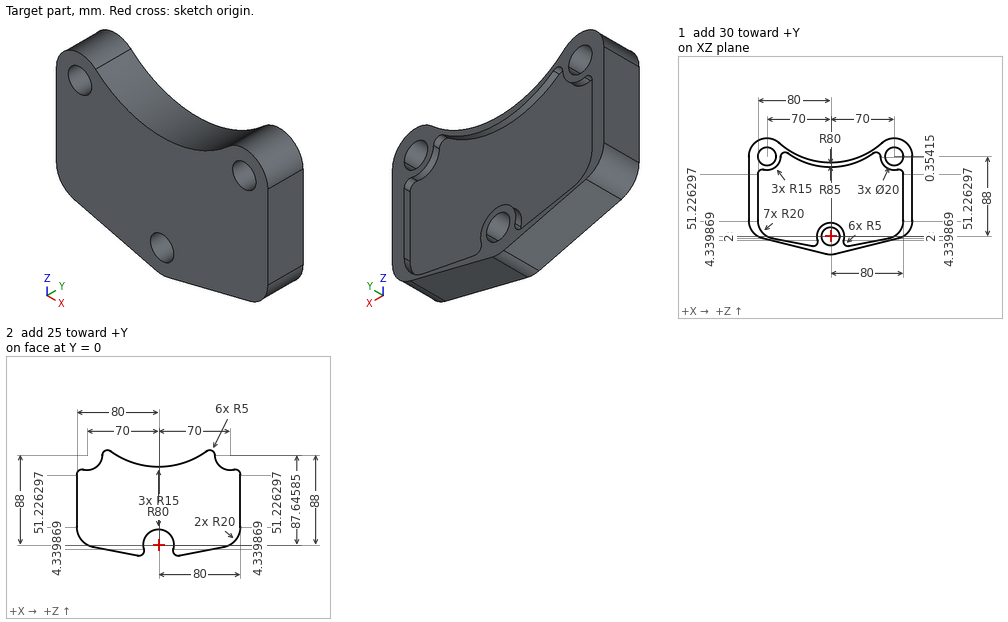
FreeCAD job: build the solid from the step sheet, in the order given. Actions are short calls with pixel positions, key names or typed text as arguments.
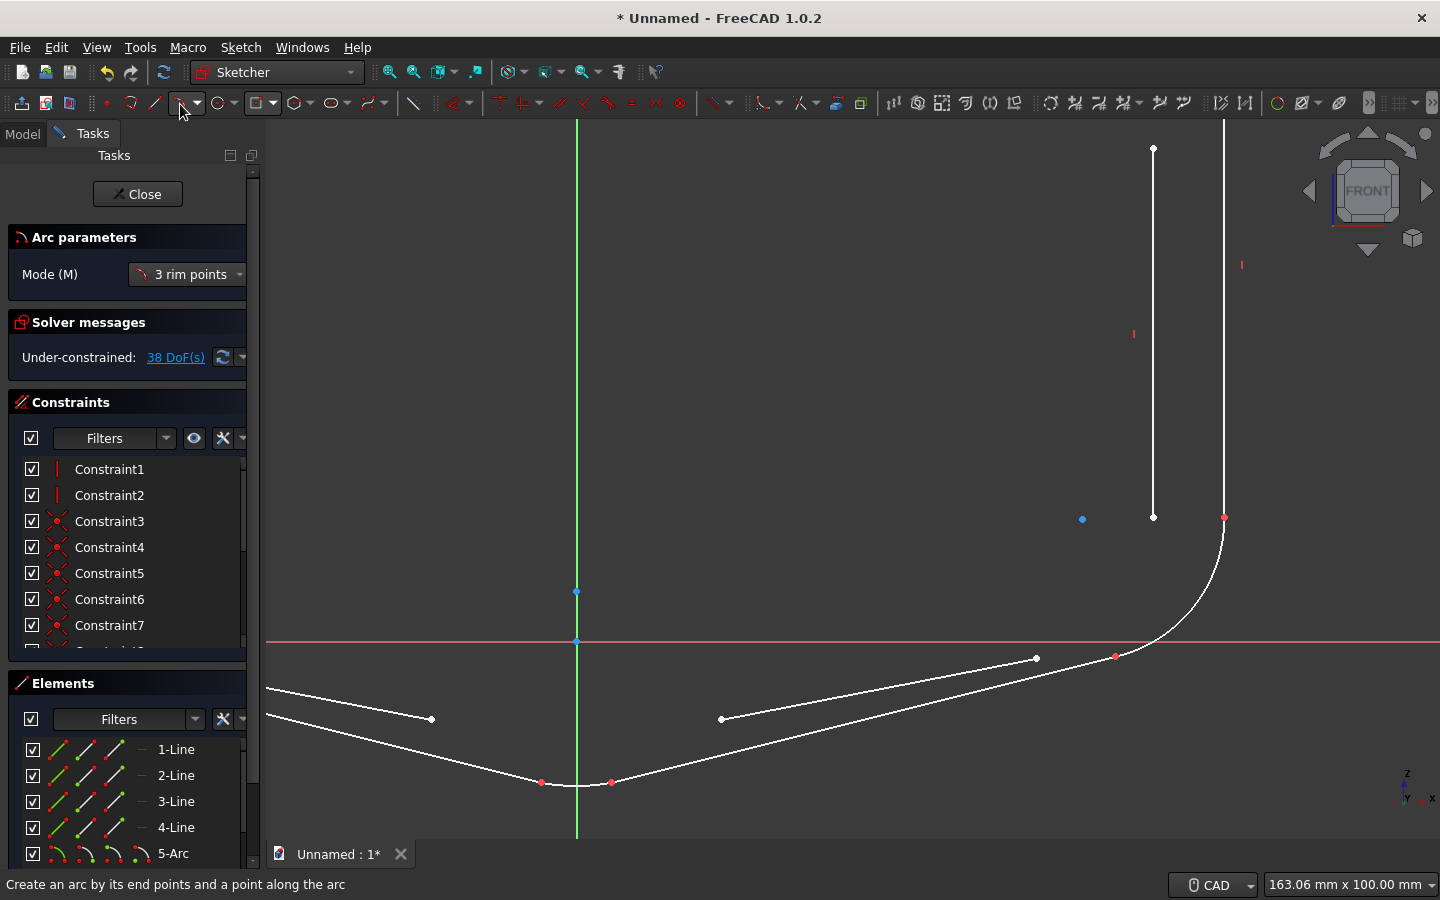
scroll(1037, 659, down, 3)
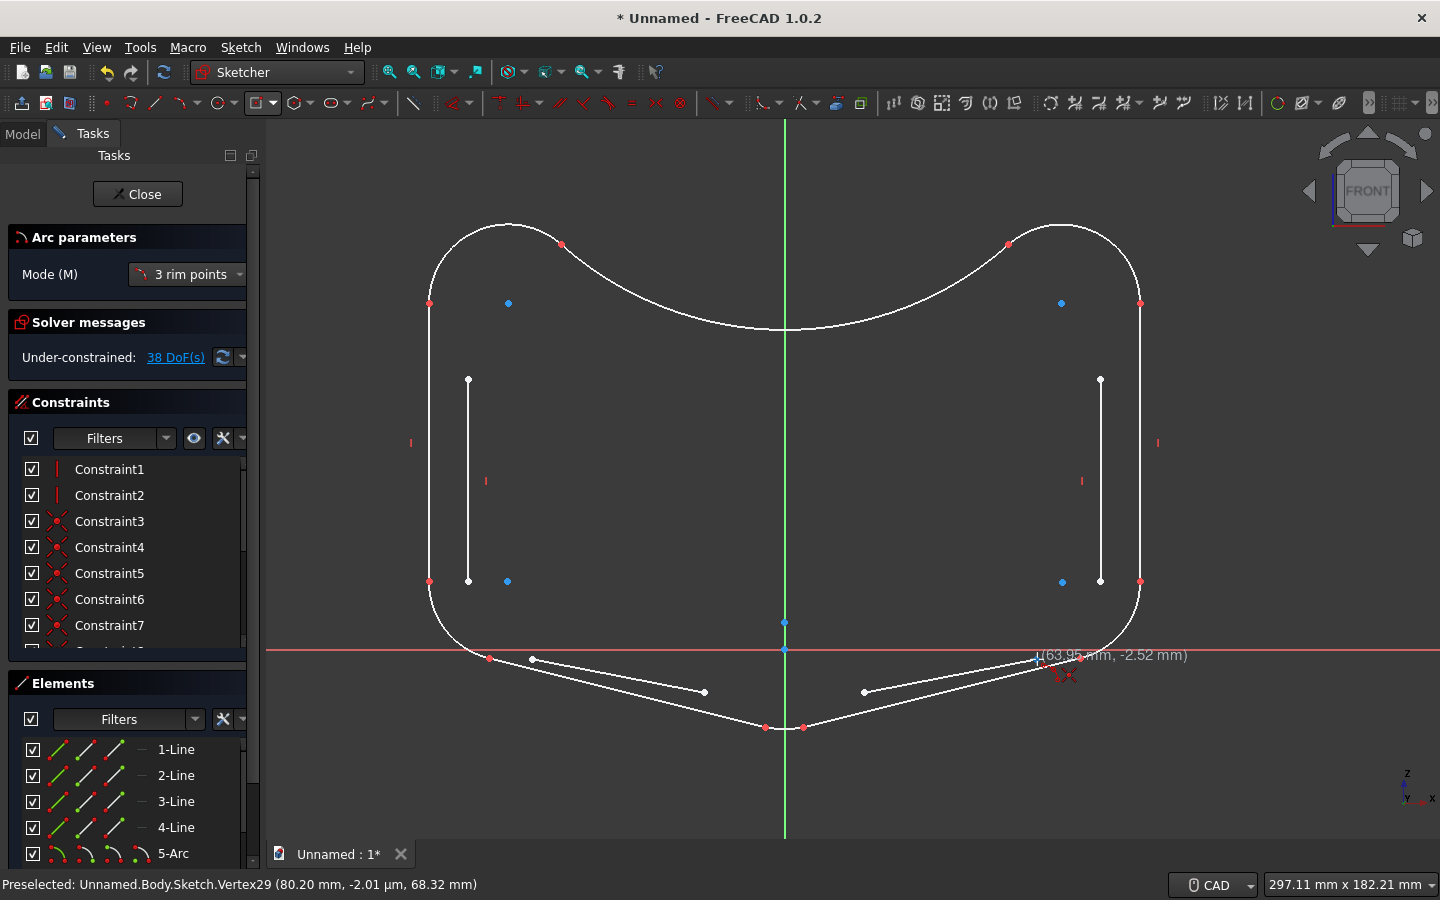
click(468, 582)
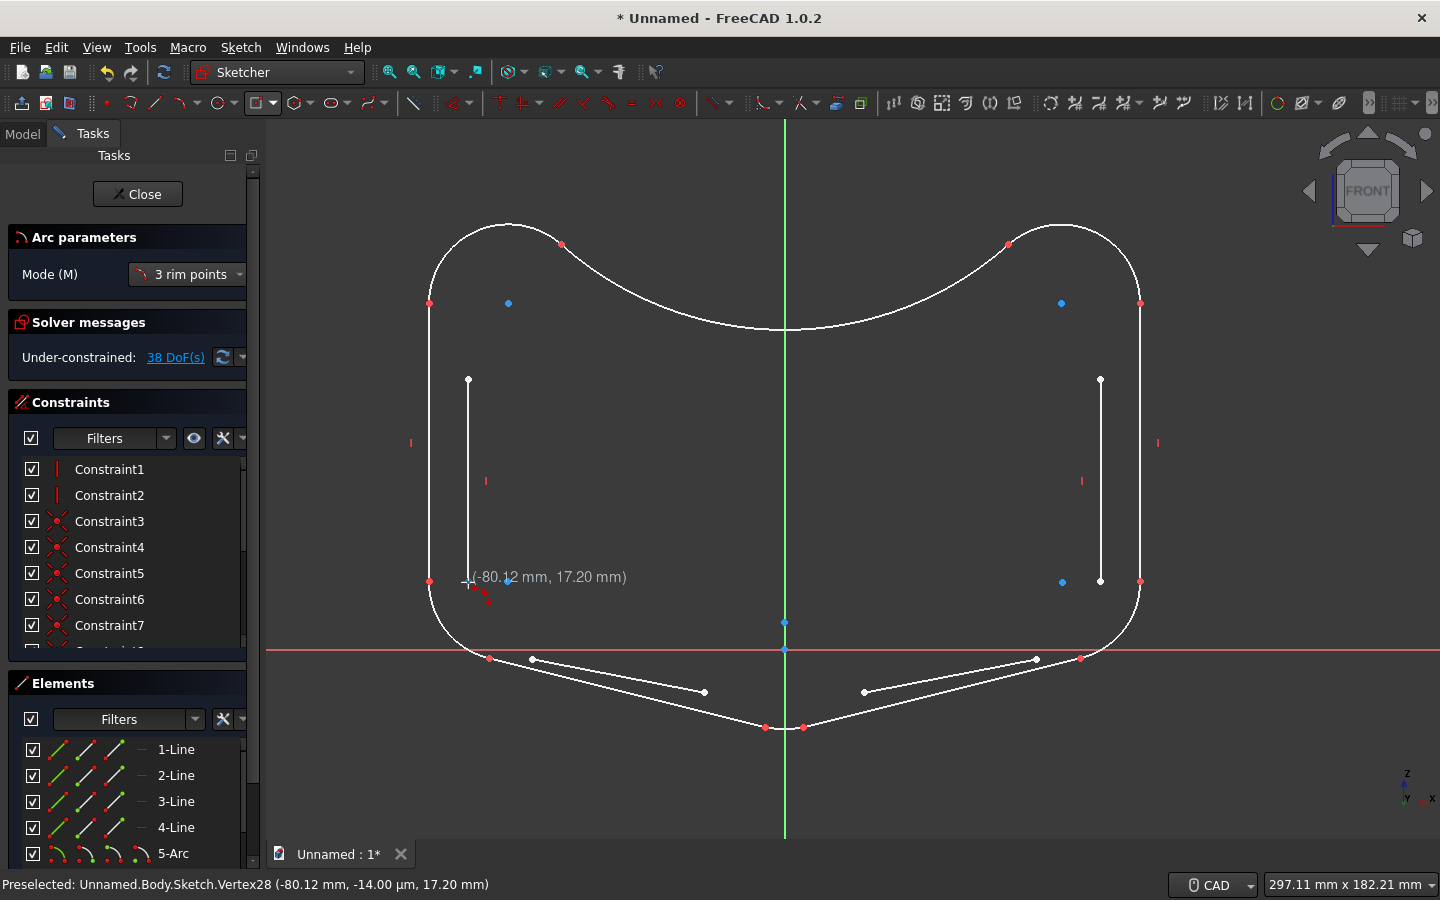
scroll(532, 659, up, 3)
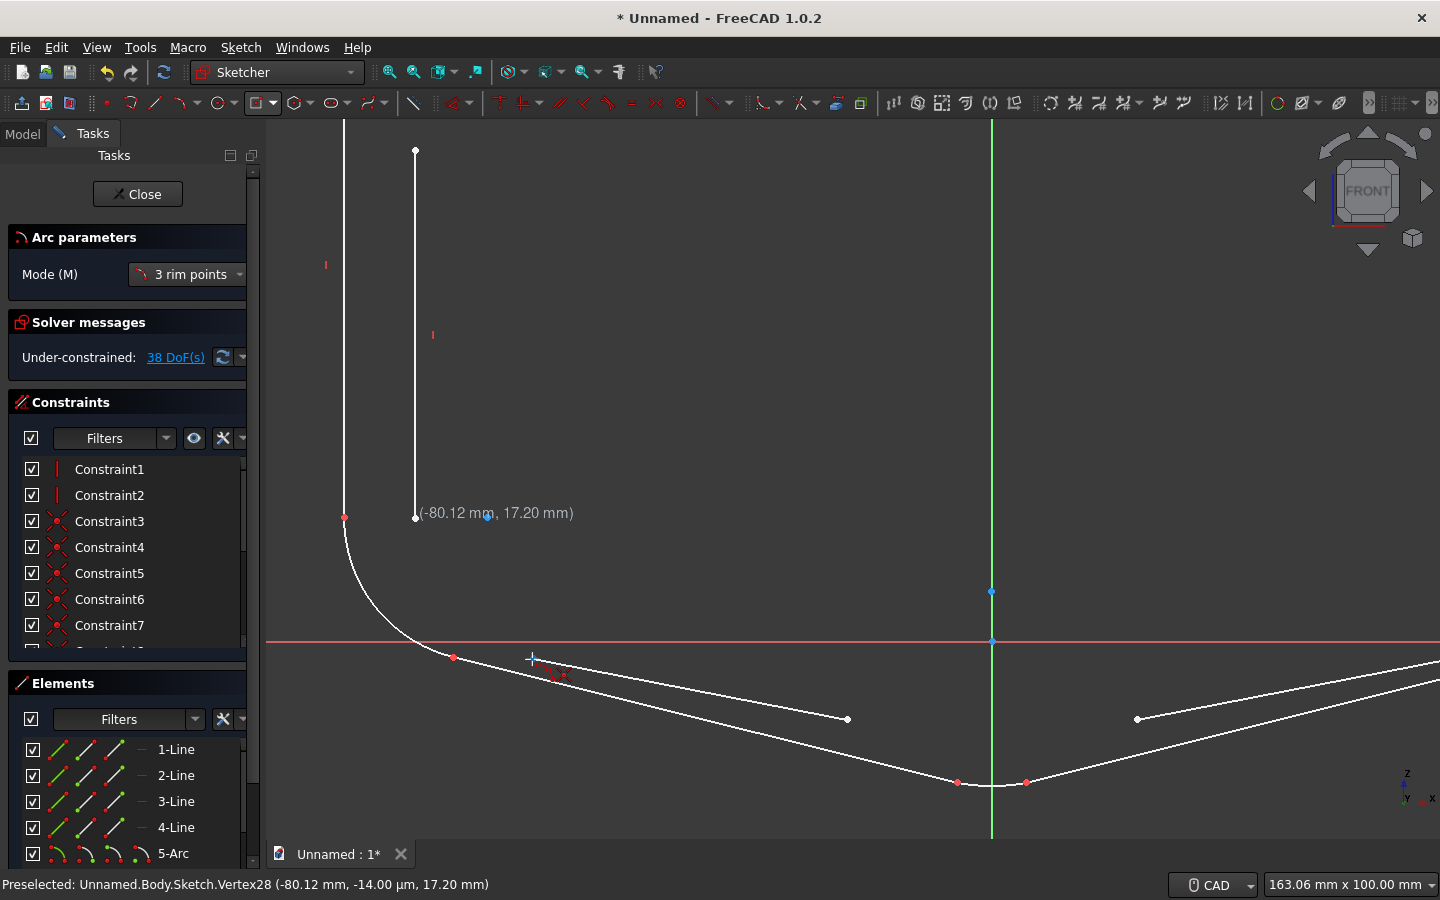
click(533, 659)
click(449, 608)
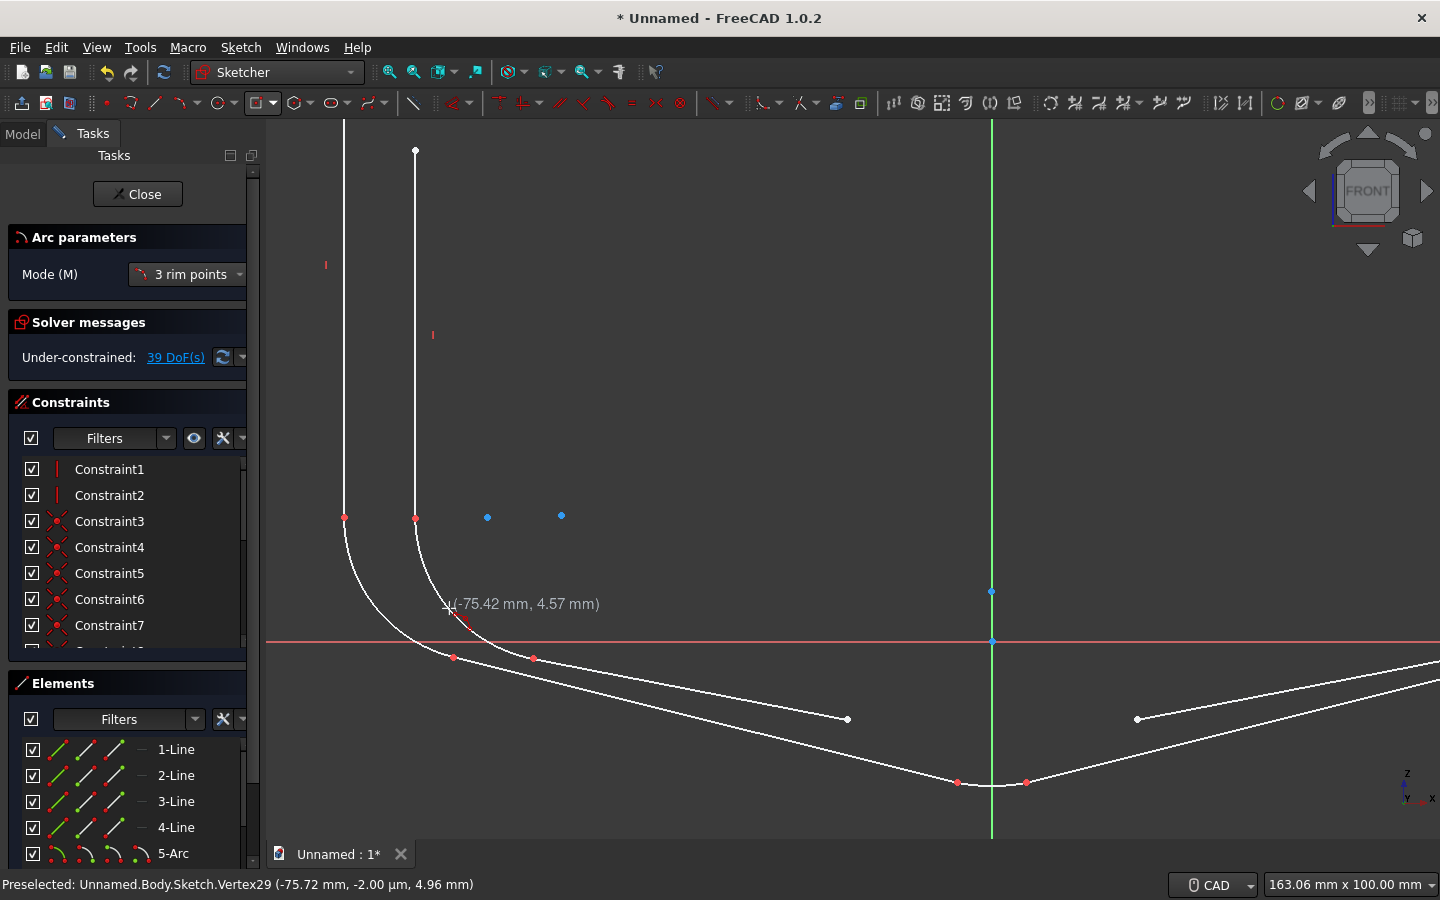
click(847, 720)
click(889, 673)
click(881, 708)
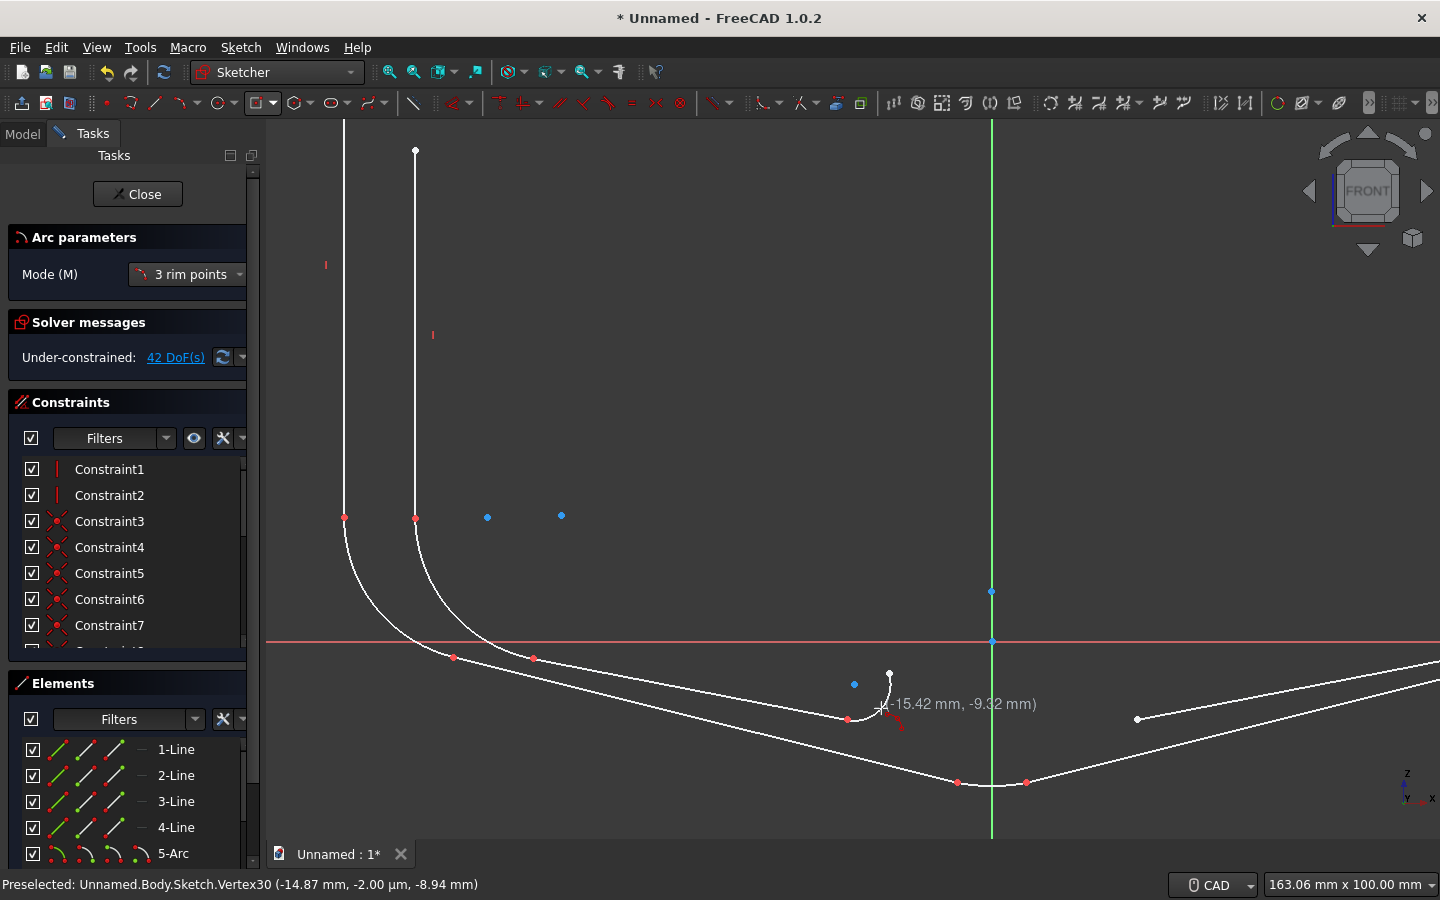
click(889, 674)
click(1095, 673)
click(1031, 541)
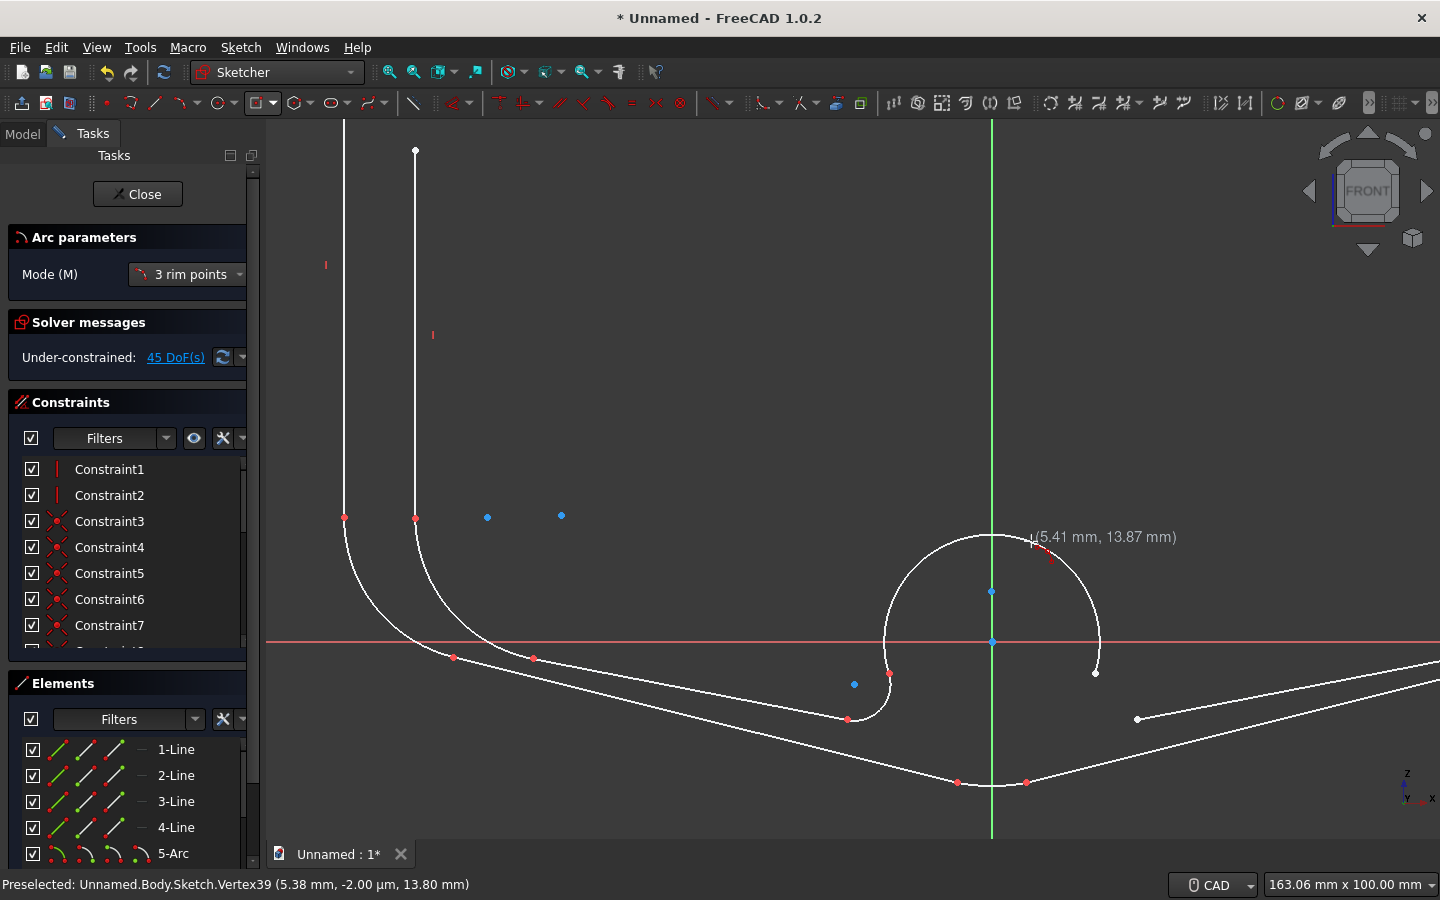
click(1095, 674)
click(1137, 720)
click(1103, 708)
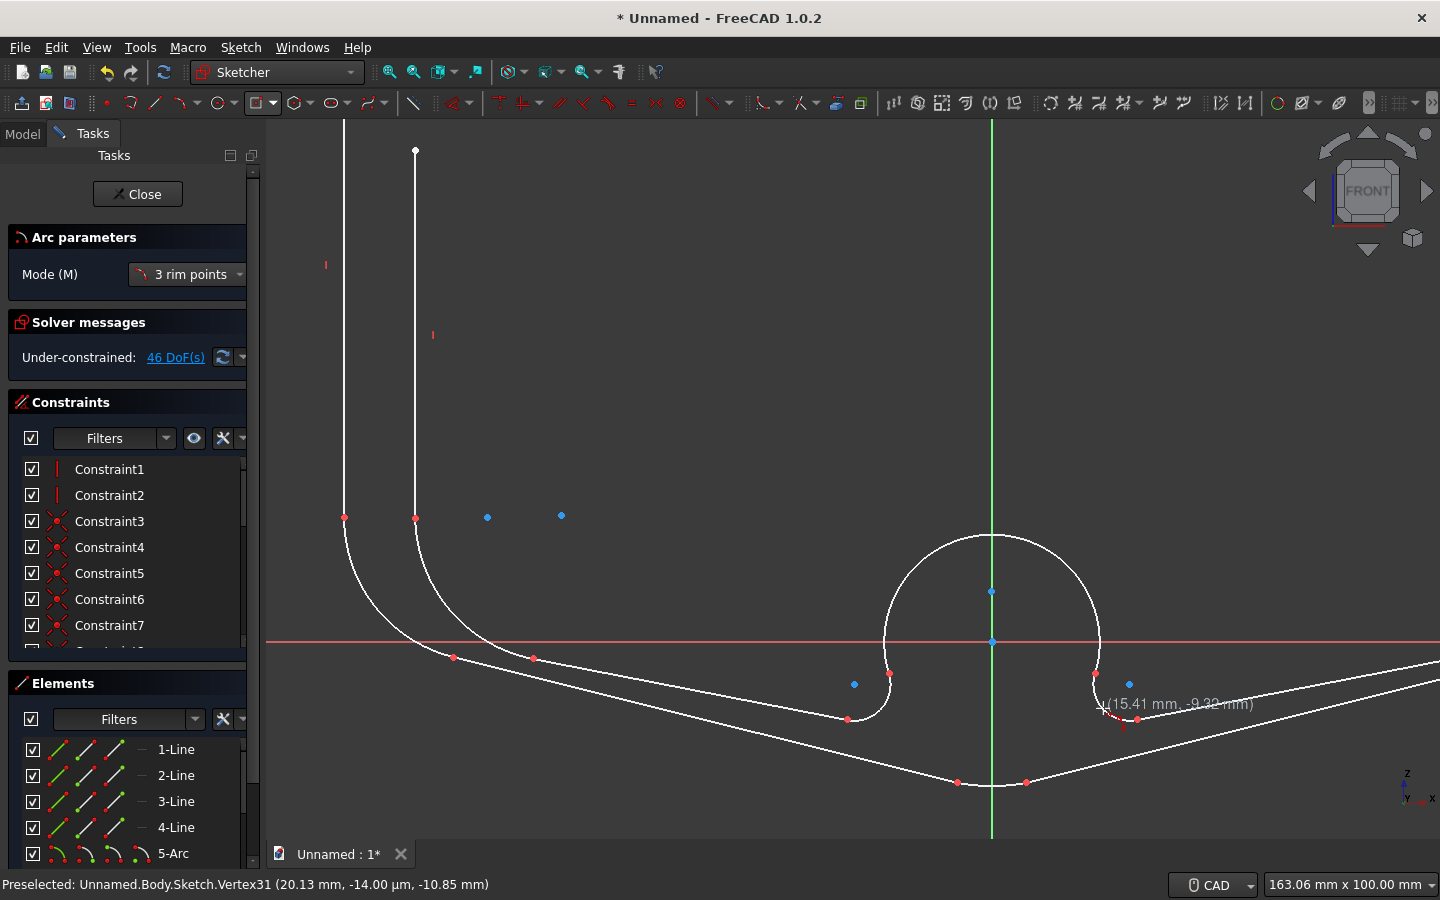
scroll(532, 659, down, 3)